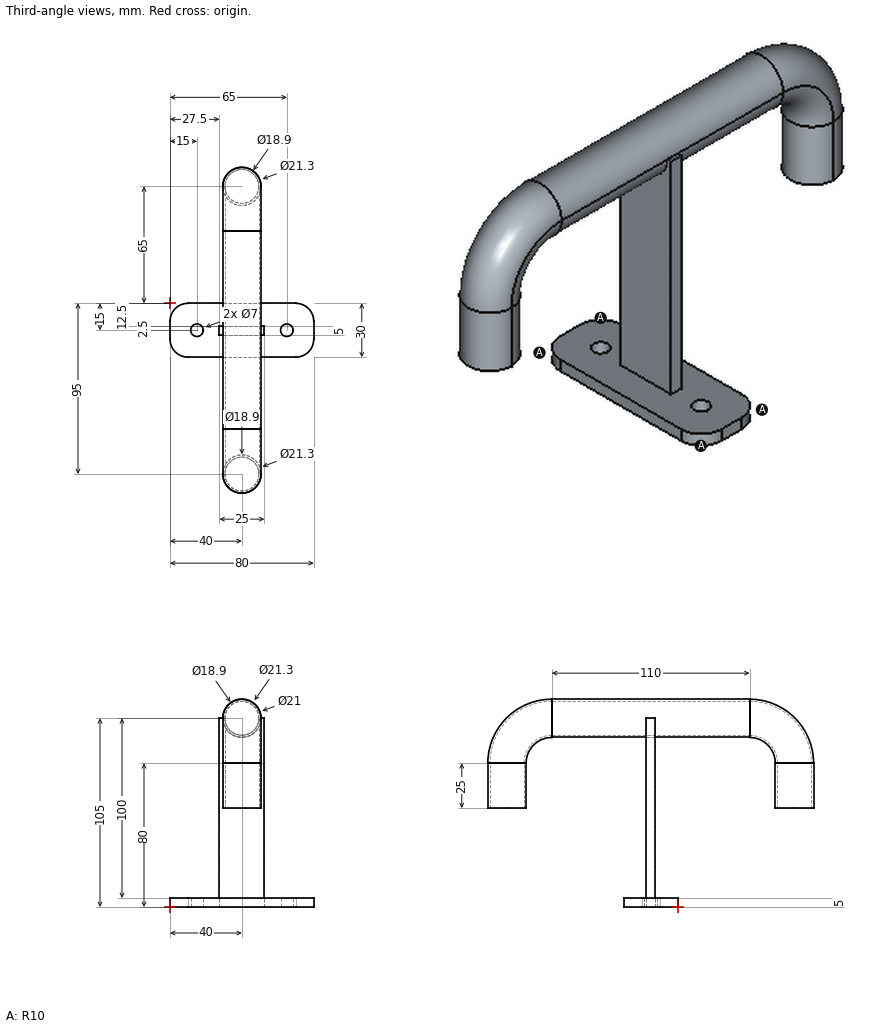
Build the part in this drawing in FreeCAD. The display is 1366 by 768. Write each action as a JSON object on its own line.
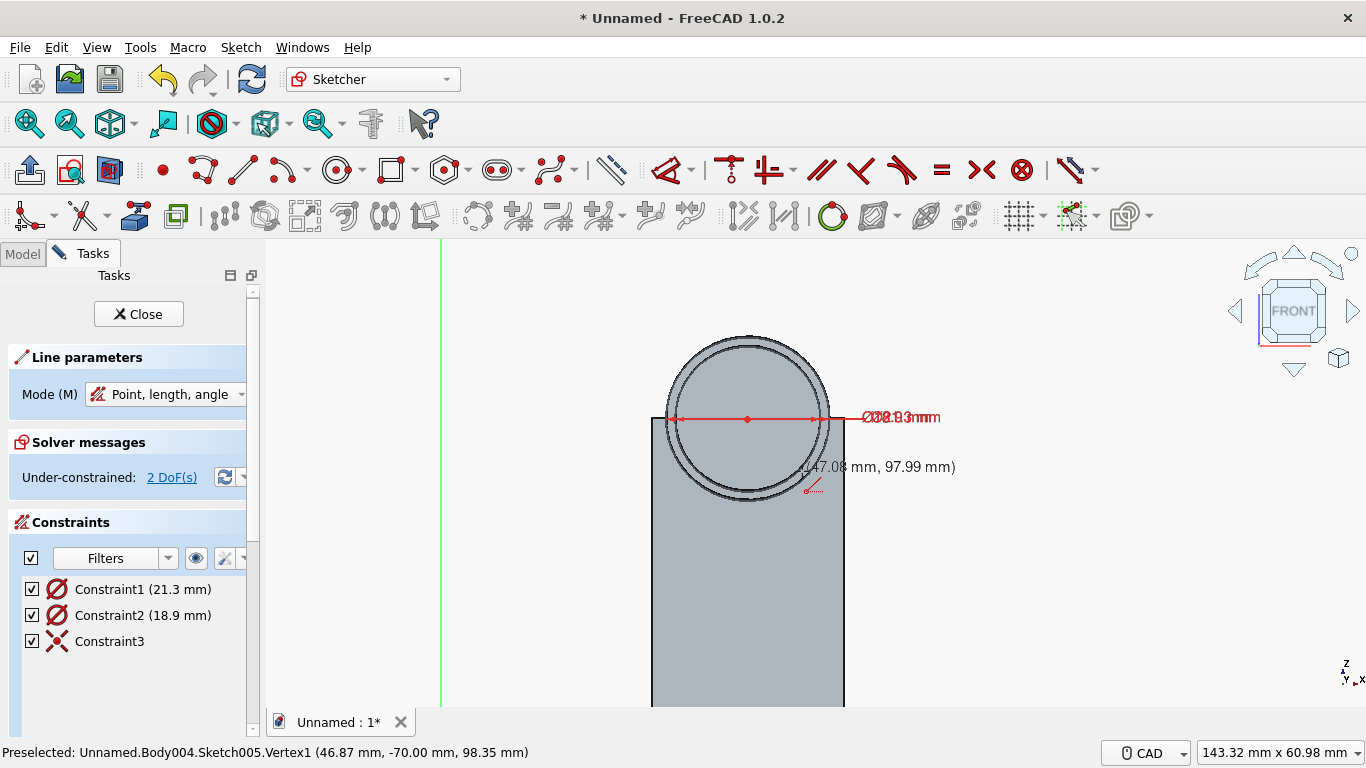
{"action": "left_click", "coordinate": [650, 610]}
{"action": "left_click", "coordinate": [846, 610]}
{"action": "key", "text": "Escape"}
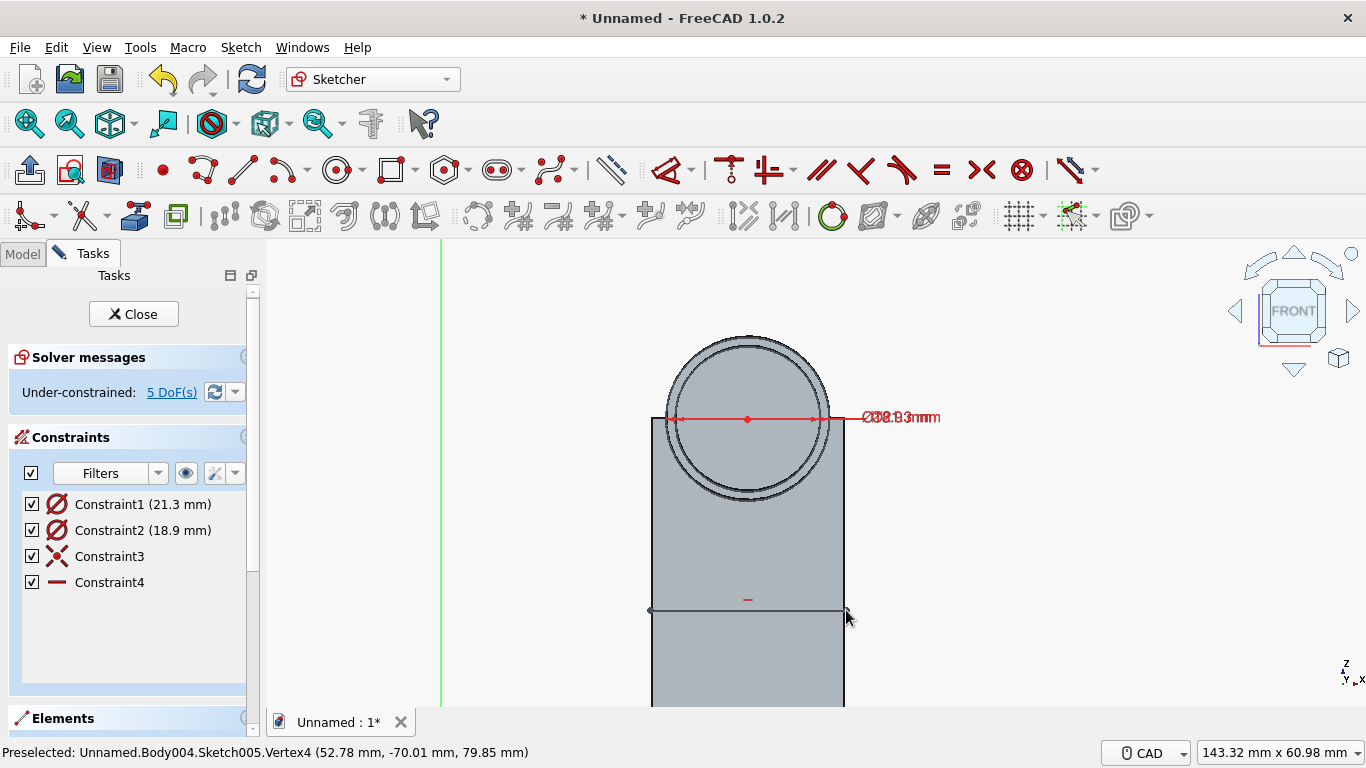
{"action": "left_click", "coordinate": [709, 611]}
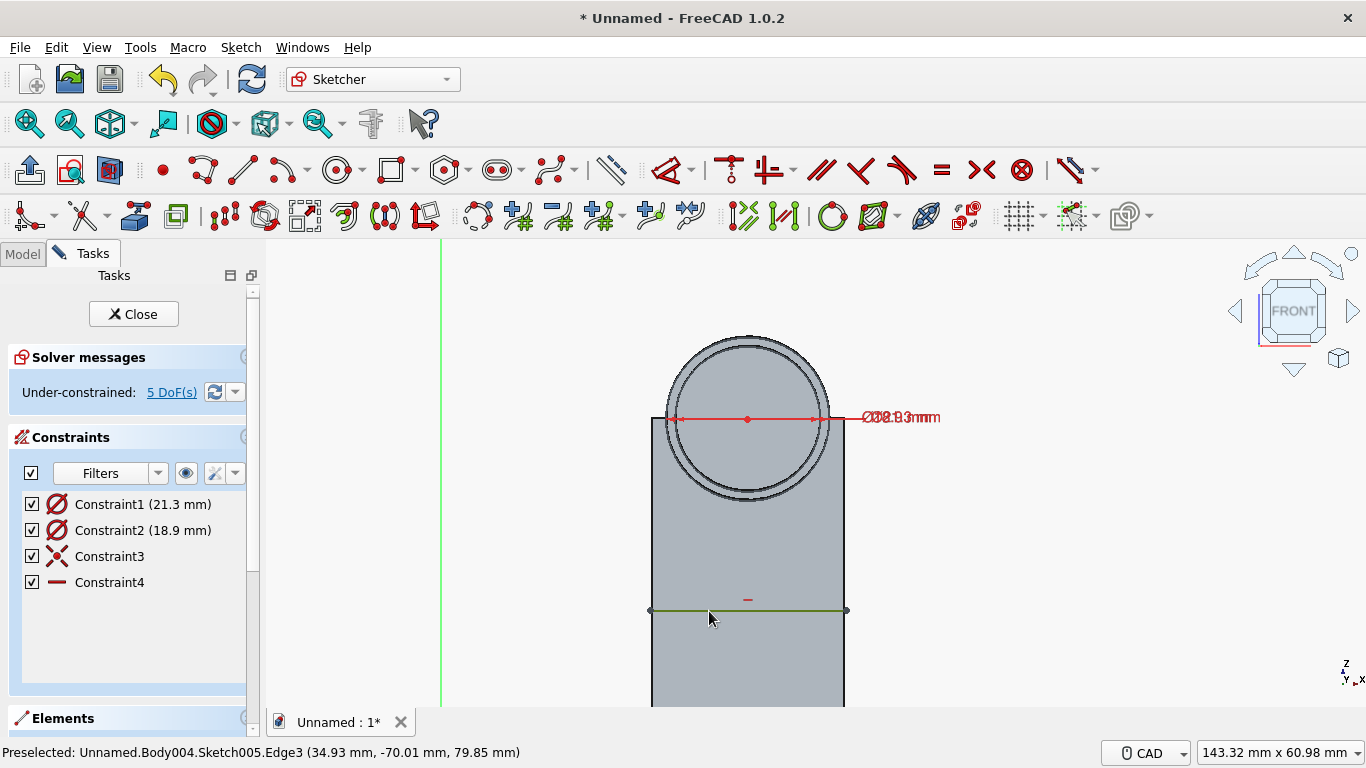
{"action": "left_click", "coordinate": [612, 170]}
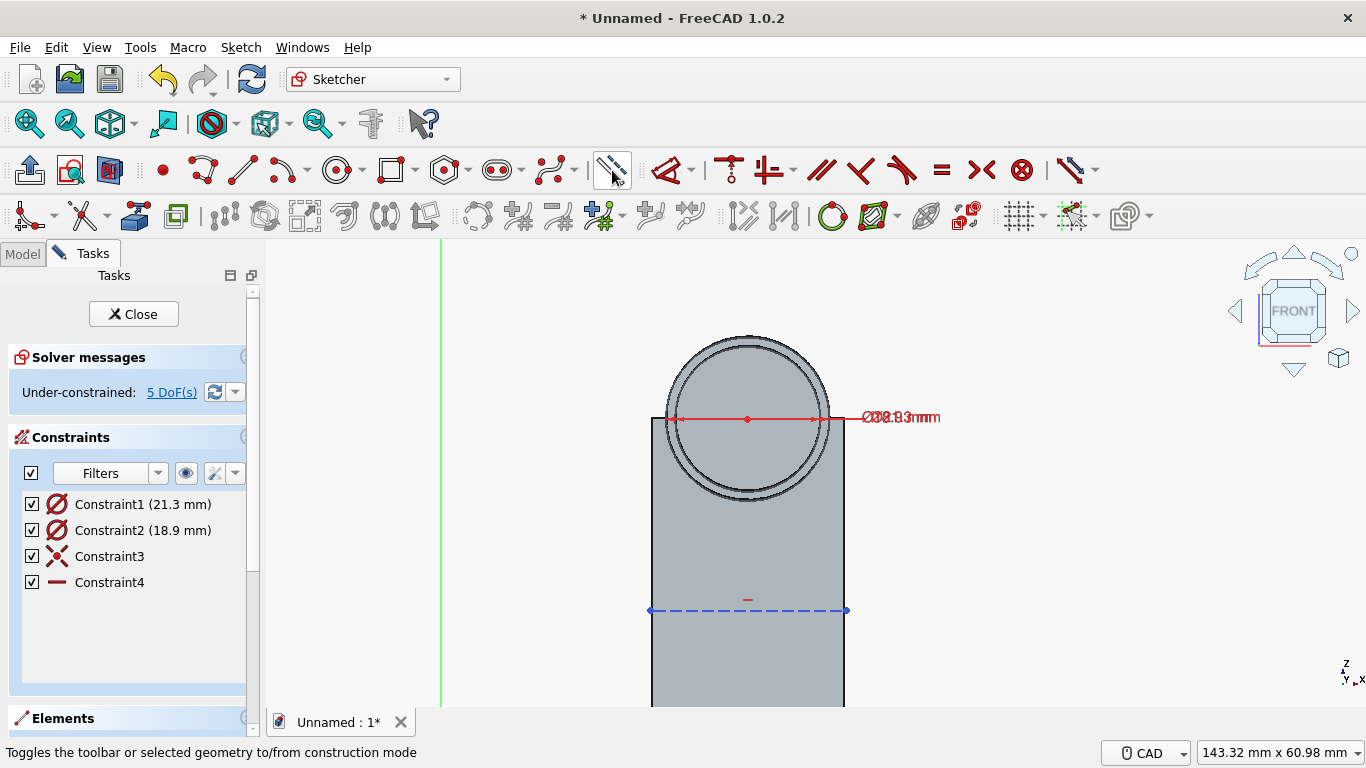
{"action": "left_click", "coordinate": [666, 170]}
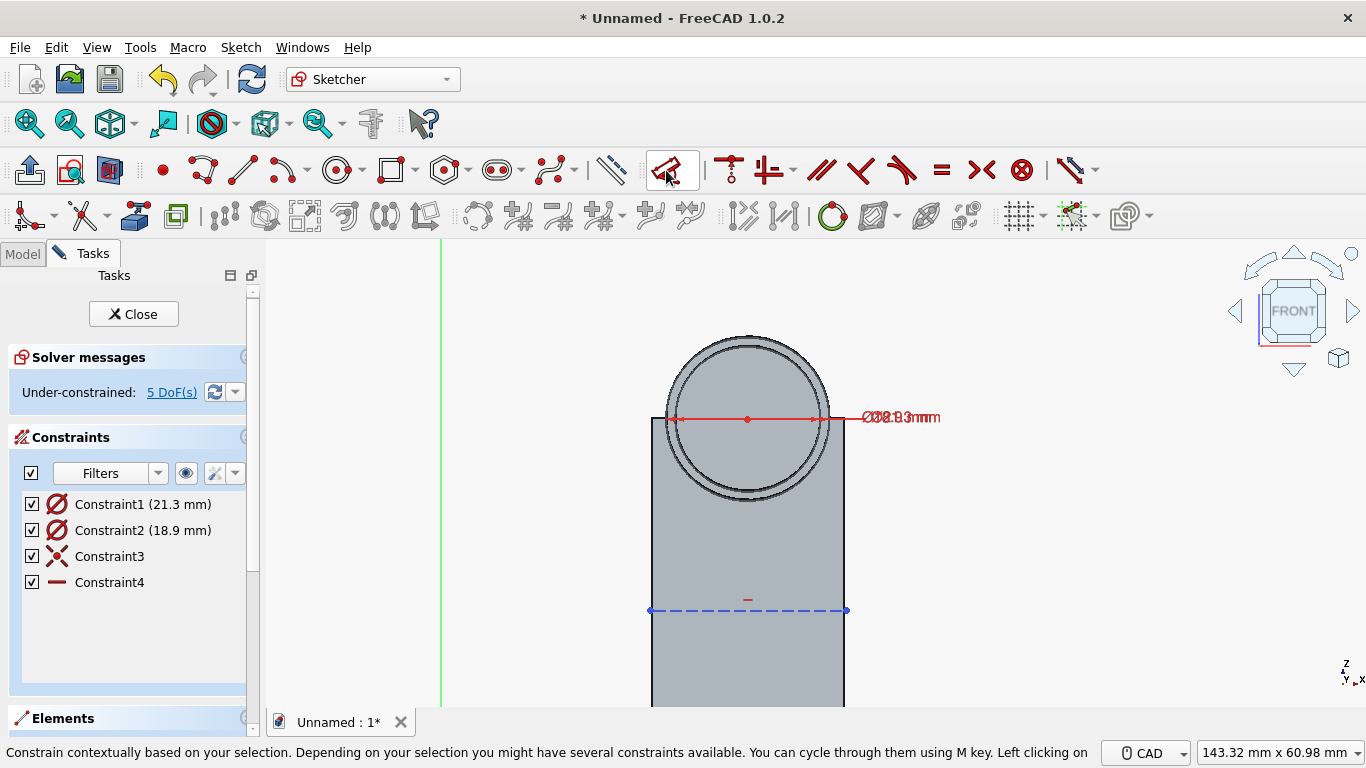
{"action": "left_click", "coordinate": [748, 419]}
{"action": "left_click", "coordinate": [594, 385]}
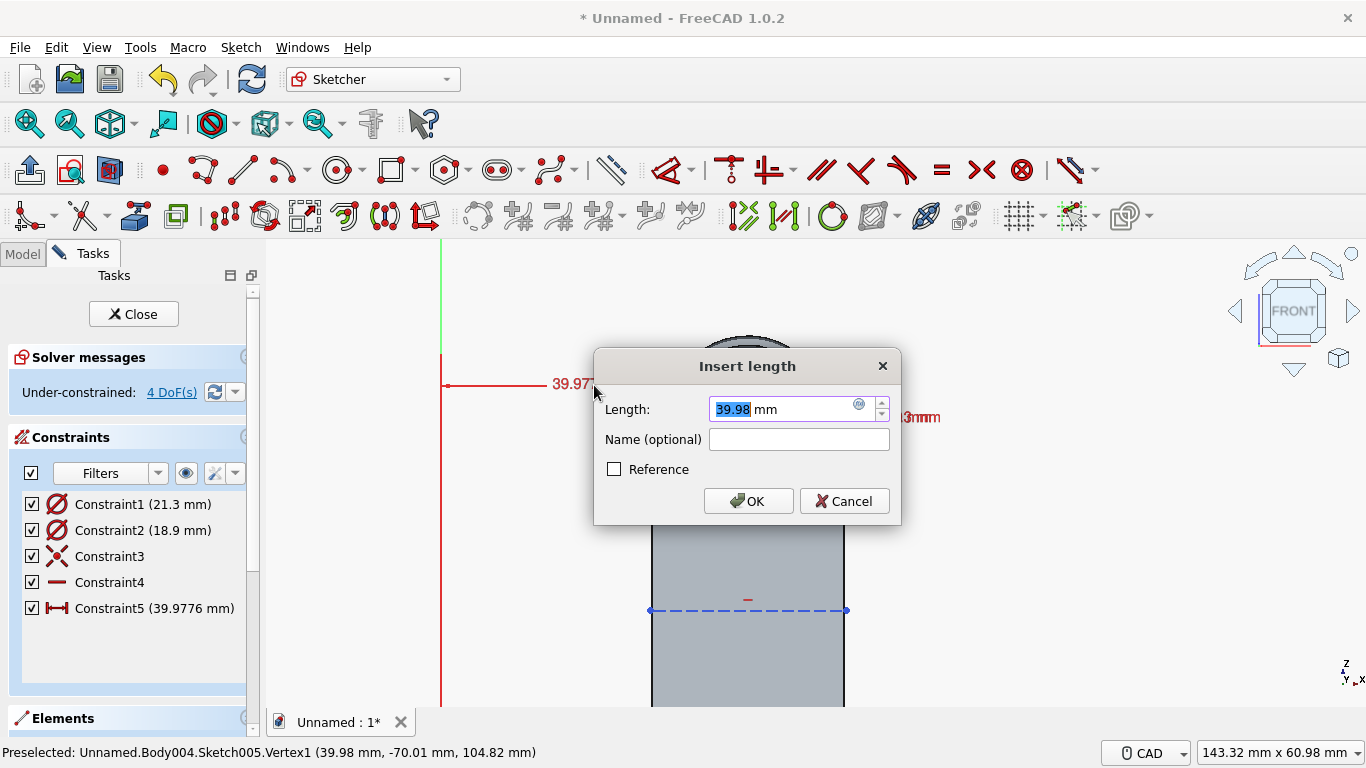
{"action": "type", "text": "40"}
{"action": "key", "text": "Return"}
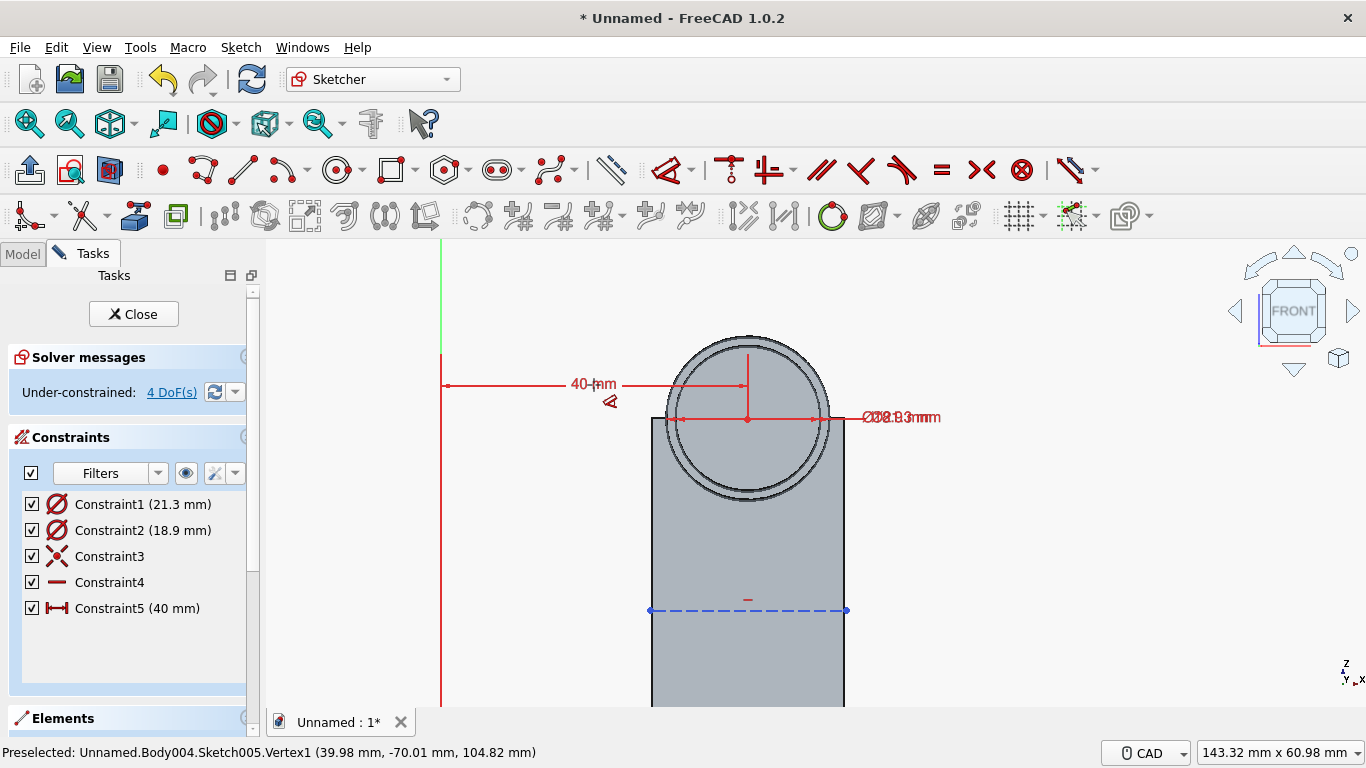
{"action": "left_click", "coordinate": [650, 611]}
{"action": "left_click", "coordinate": [407, 645]}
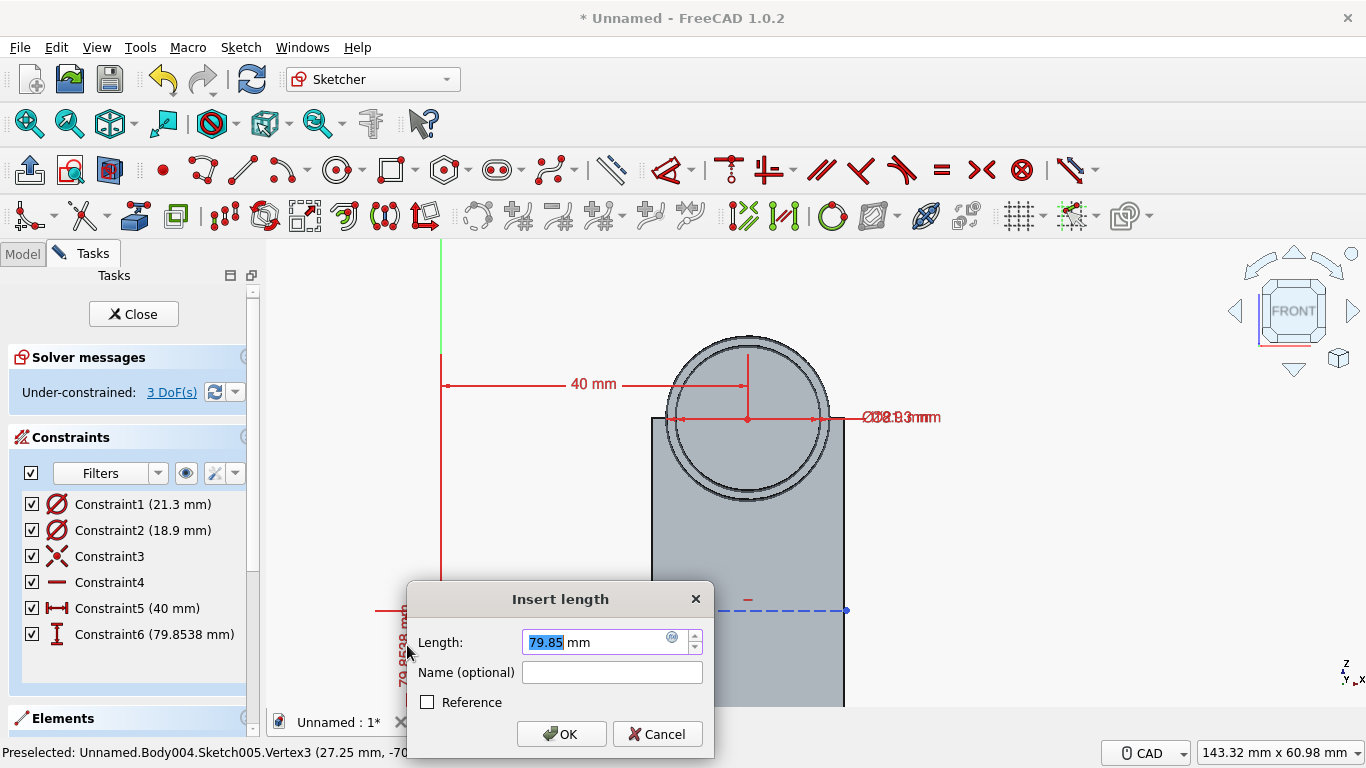
{"action": "type", "text": "80"}
{"action": "key", "text": "Return"}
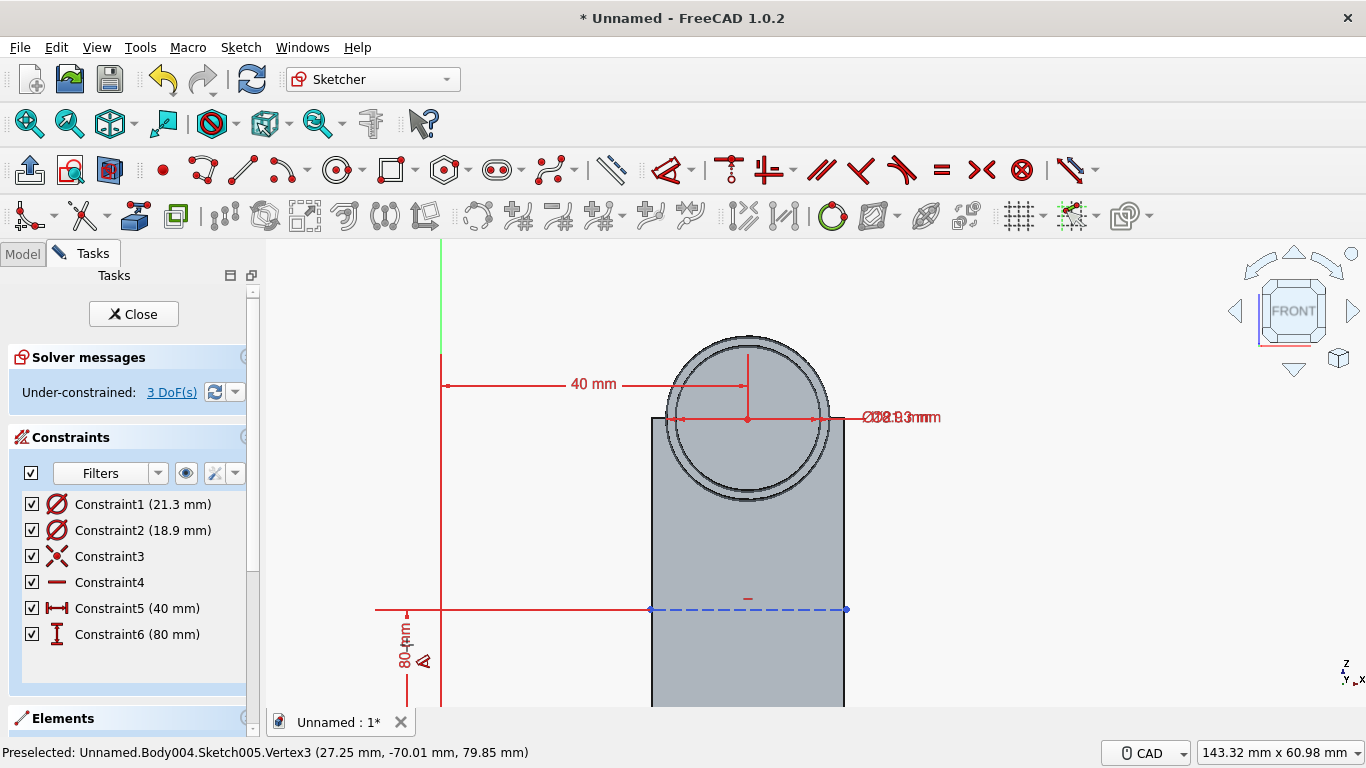
{"action": "left_click", "coordinate": [748, 419]}
{"action": "left_click", "coordinate": [407, 549]}